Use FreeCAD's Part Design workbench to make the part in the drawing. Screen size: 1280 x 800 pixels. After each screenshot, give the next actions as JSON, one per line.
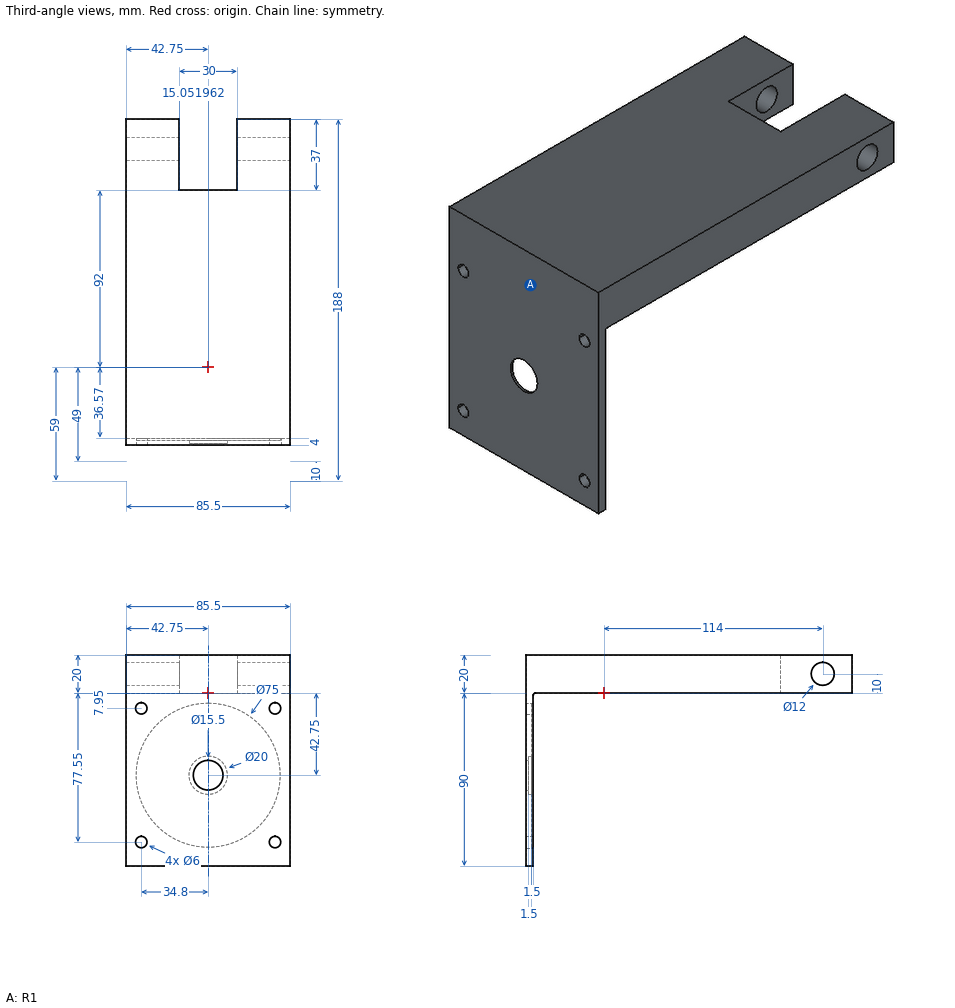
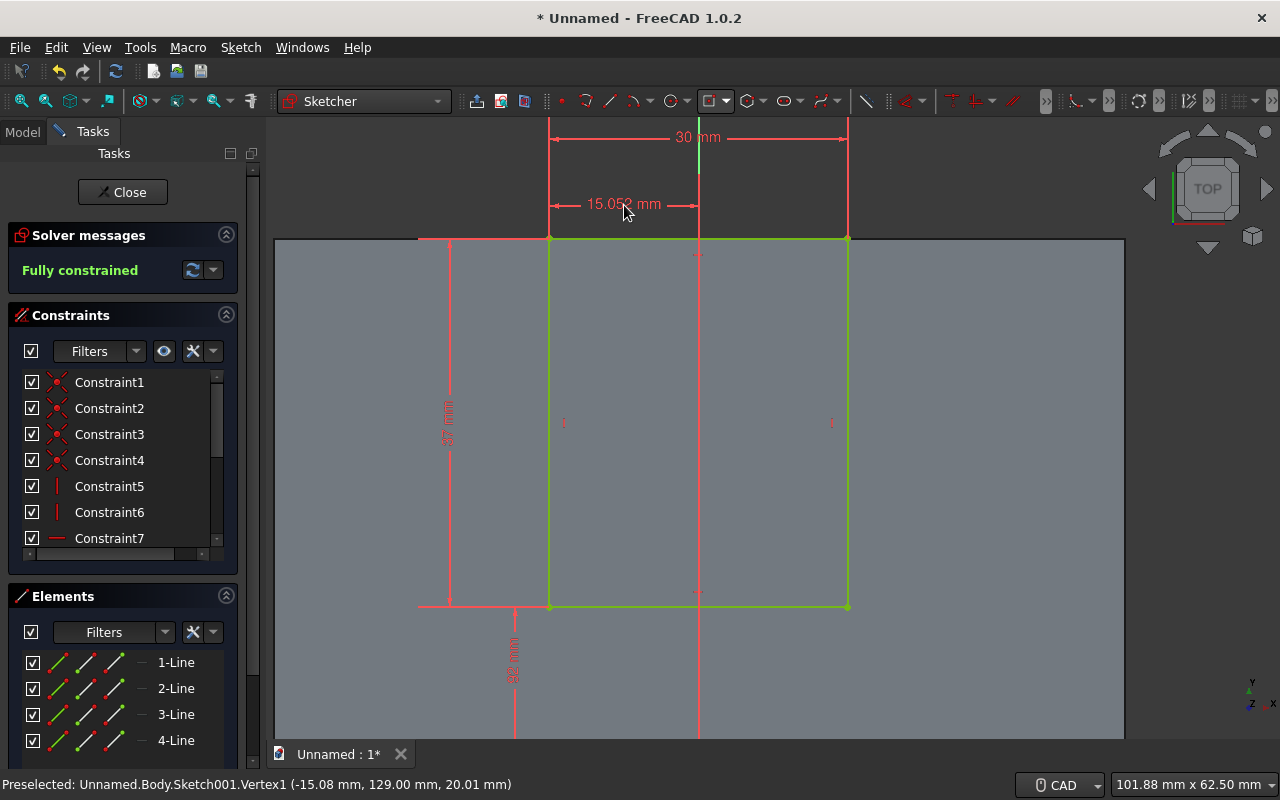
{"action": "left_click", "coordinate": [123, 192]}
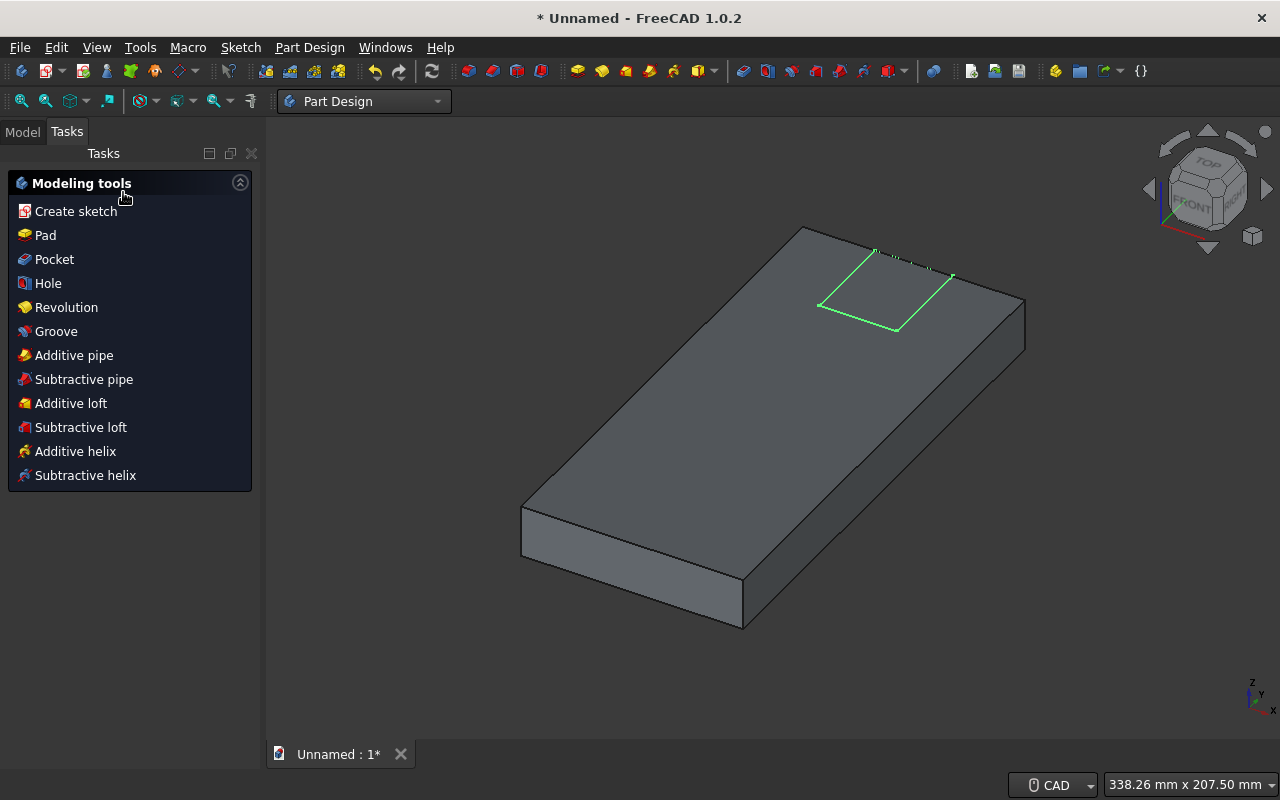
{"action": "left_click", "coordinate": [744, 72]}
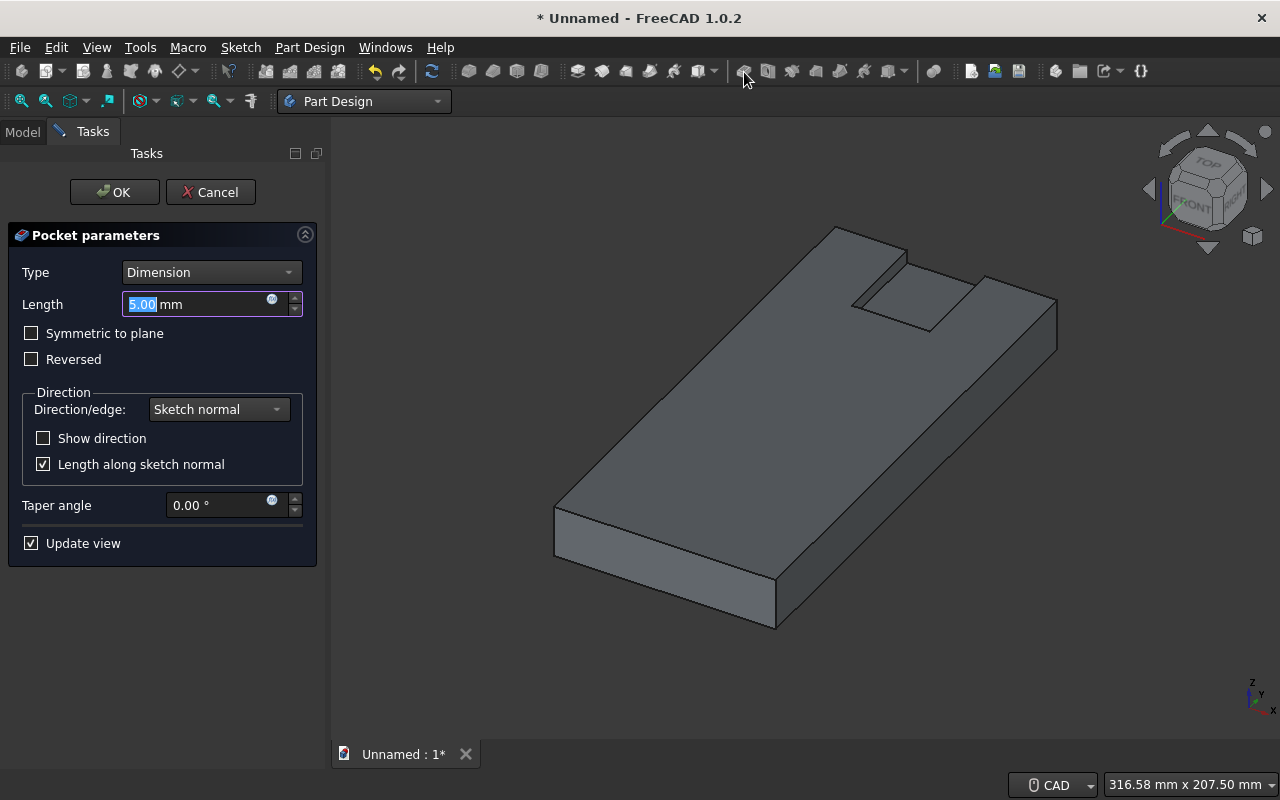
{"action": "type", "text": "20"}
{"action": "key", "text": "Tab"}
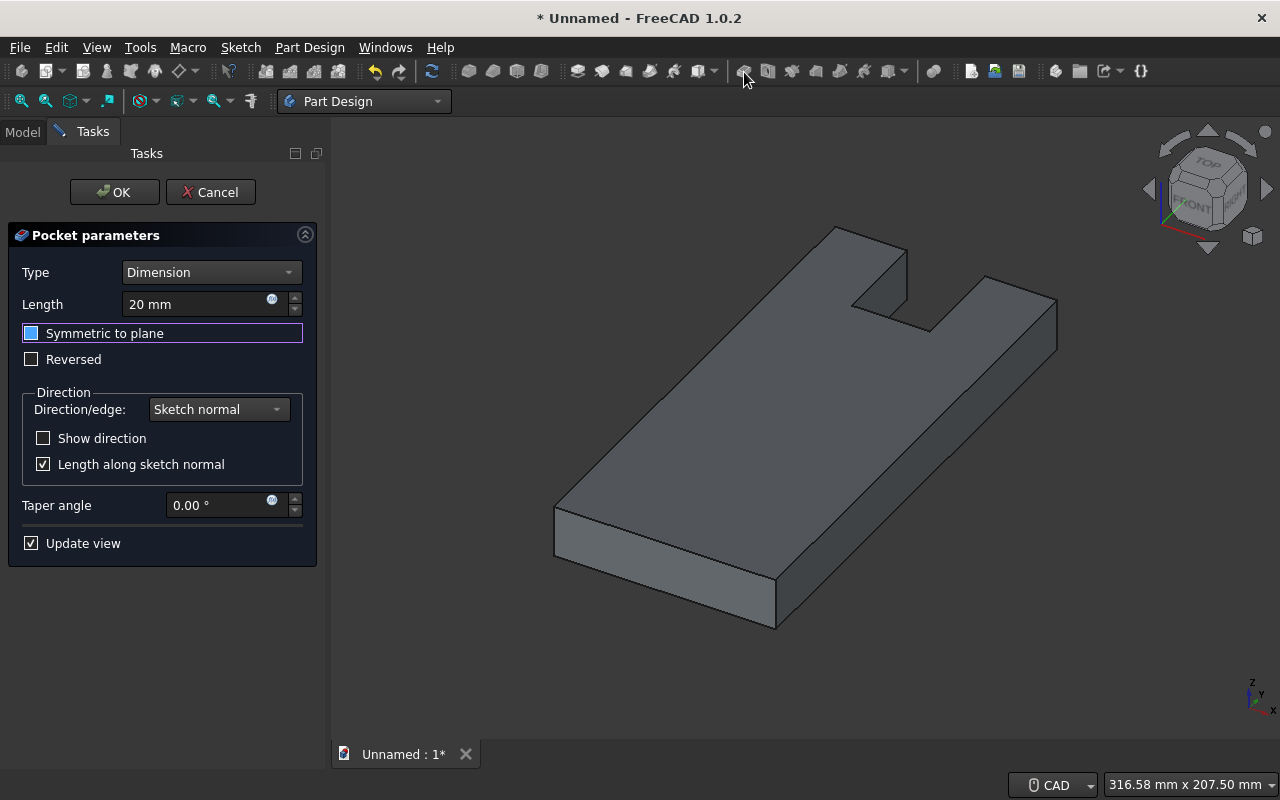
{"action": "left_click", "coordinate": [115, 192]}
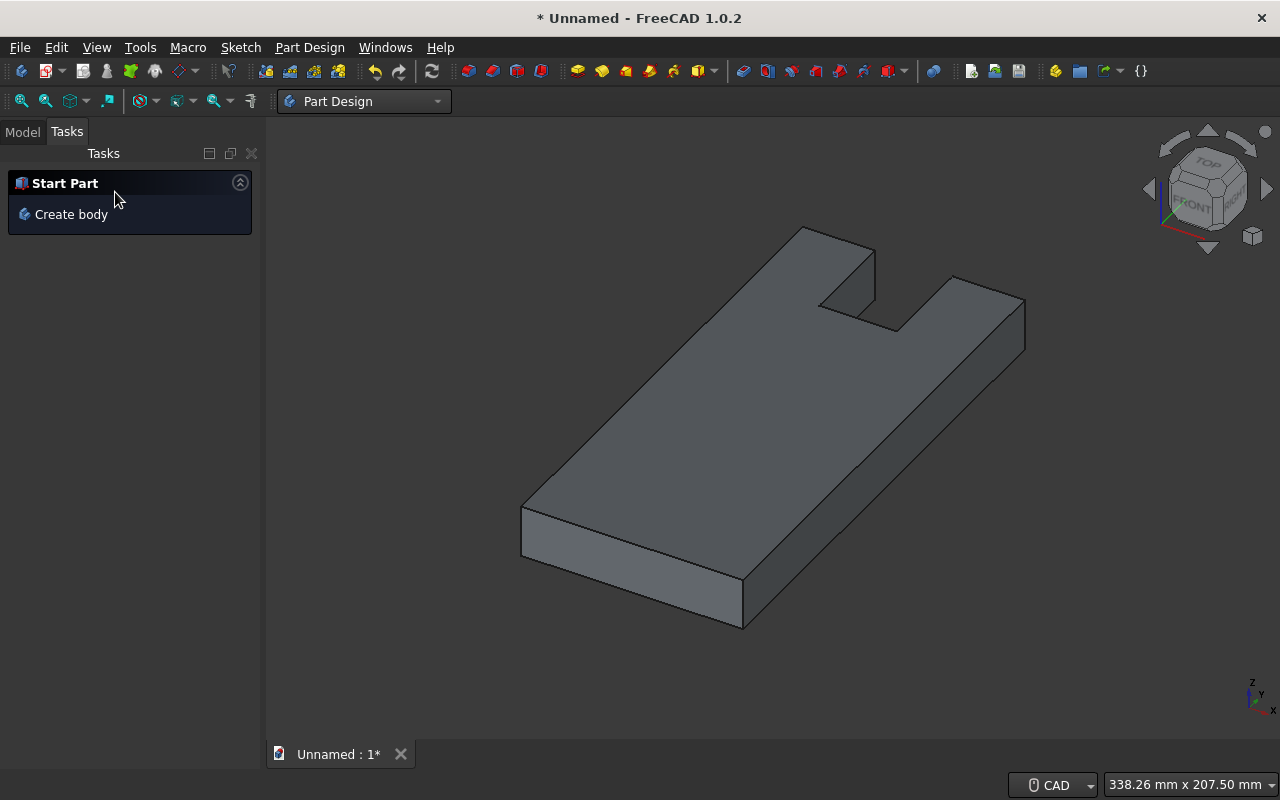
{"action": "key", "text": "6"}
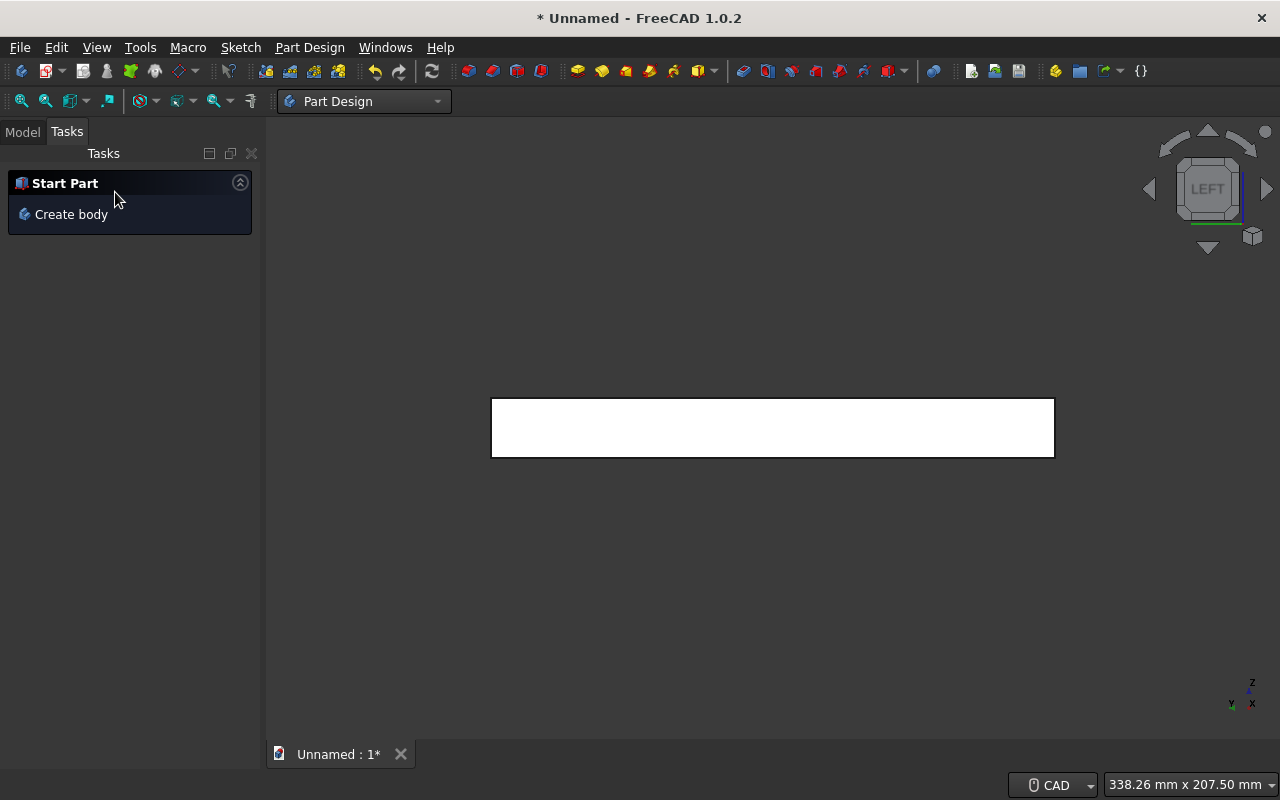
{"action": "left_click", "coordinate": [531, 427]}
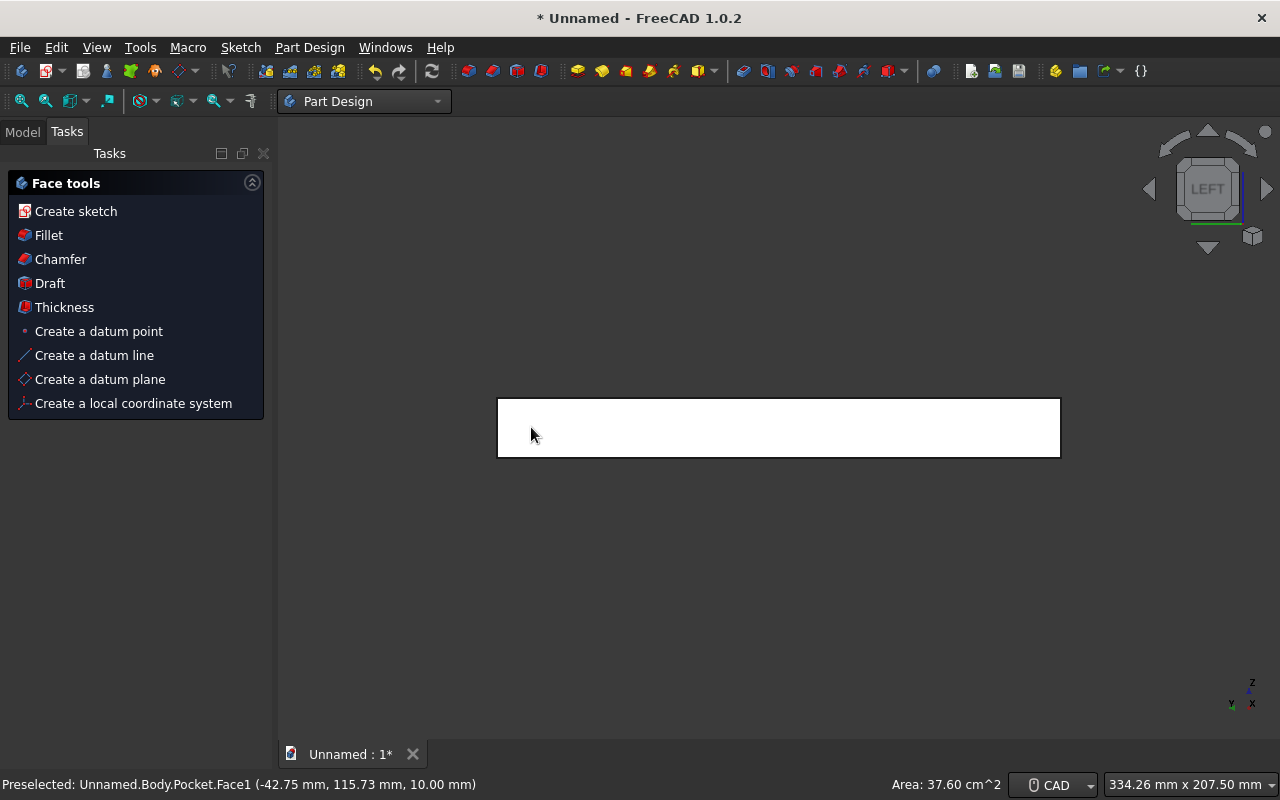
{"action": "left_click", "coordinate": [46, 72]}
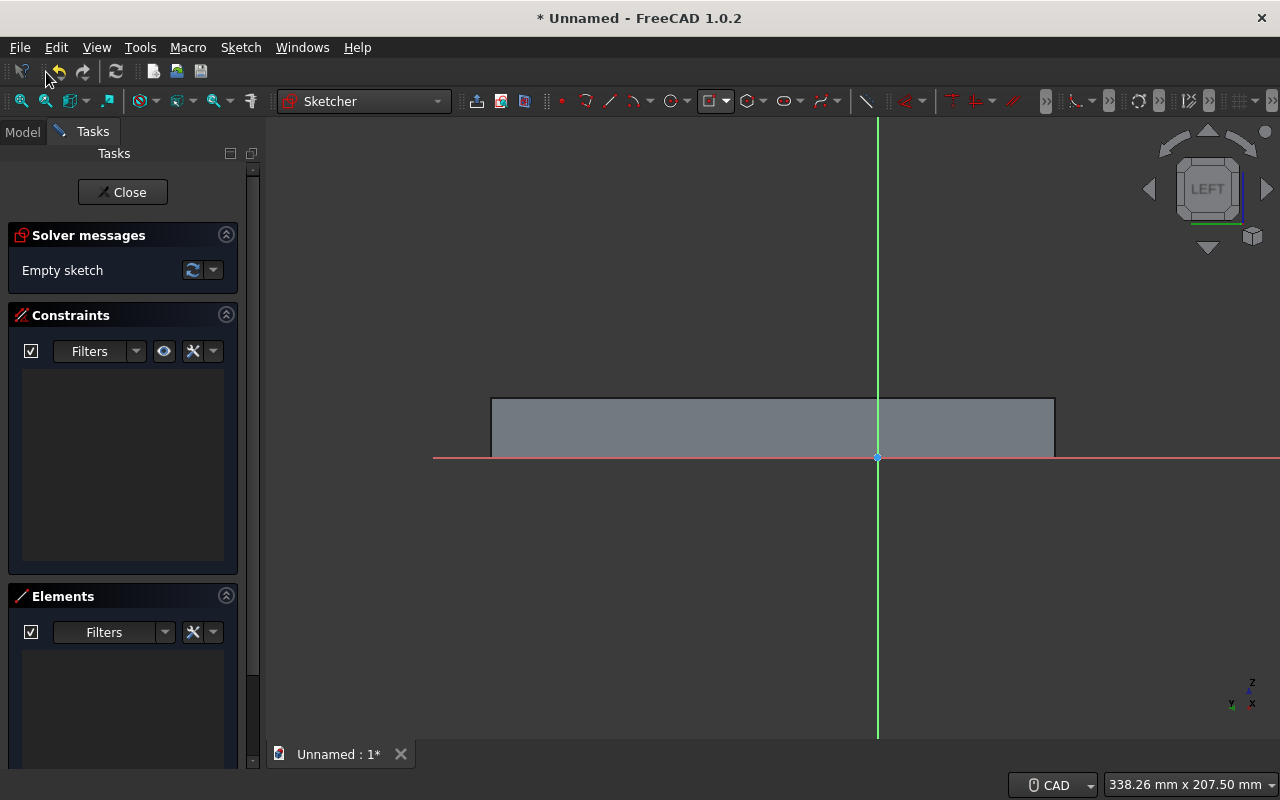
{"action": "scroll", "coordinate": [519, 428], "scroll_direction": "up", "scroll_amount": 12}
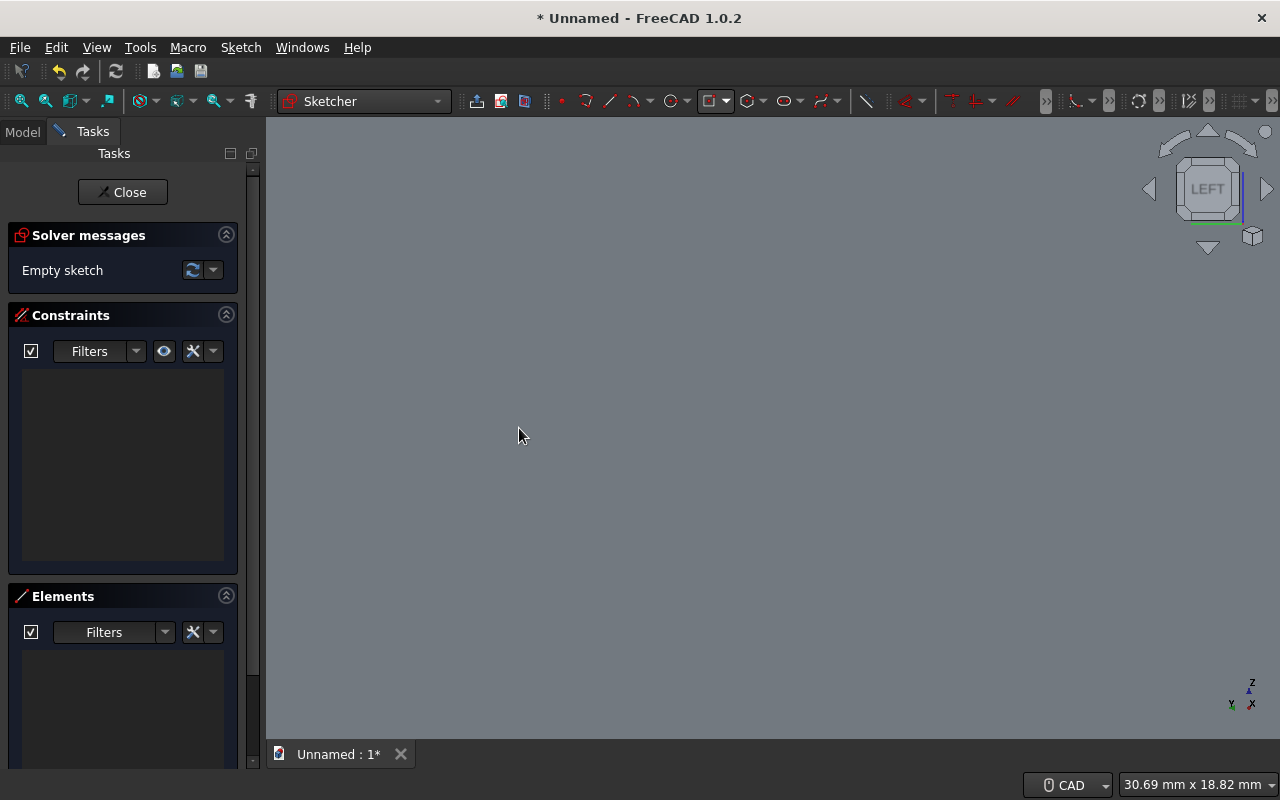
{"action": "left_click", "coordinate": [672, 102]}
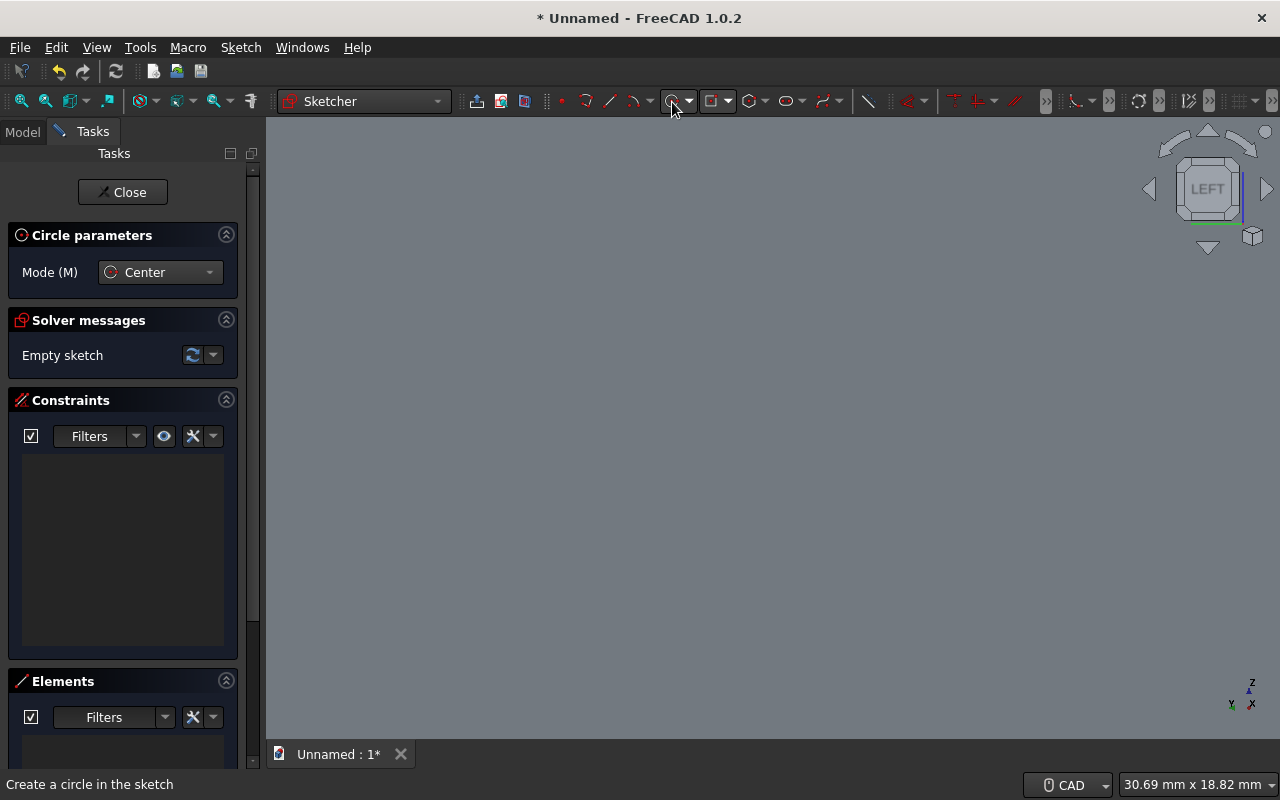
{"action": "left_click", "coordinate": [706, 423]}
{"action": "mouse_move", "coordinate": [846, 283]}